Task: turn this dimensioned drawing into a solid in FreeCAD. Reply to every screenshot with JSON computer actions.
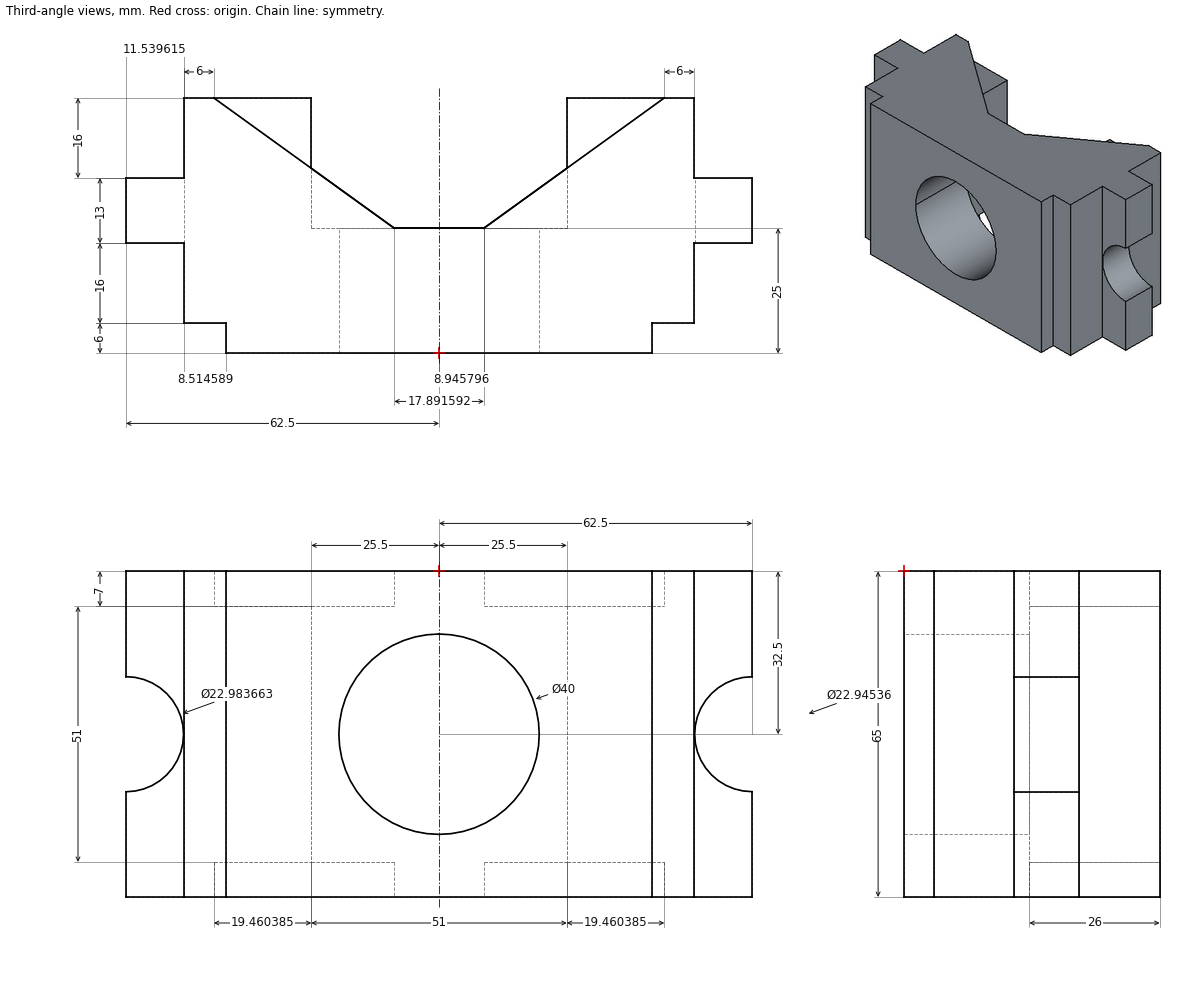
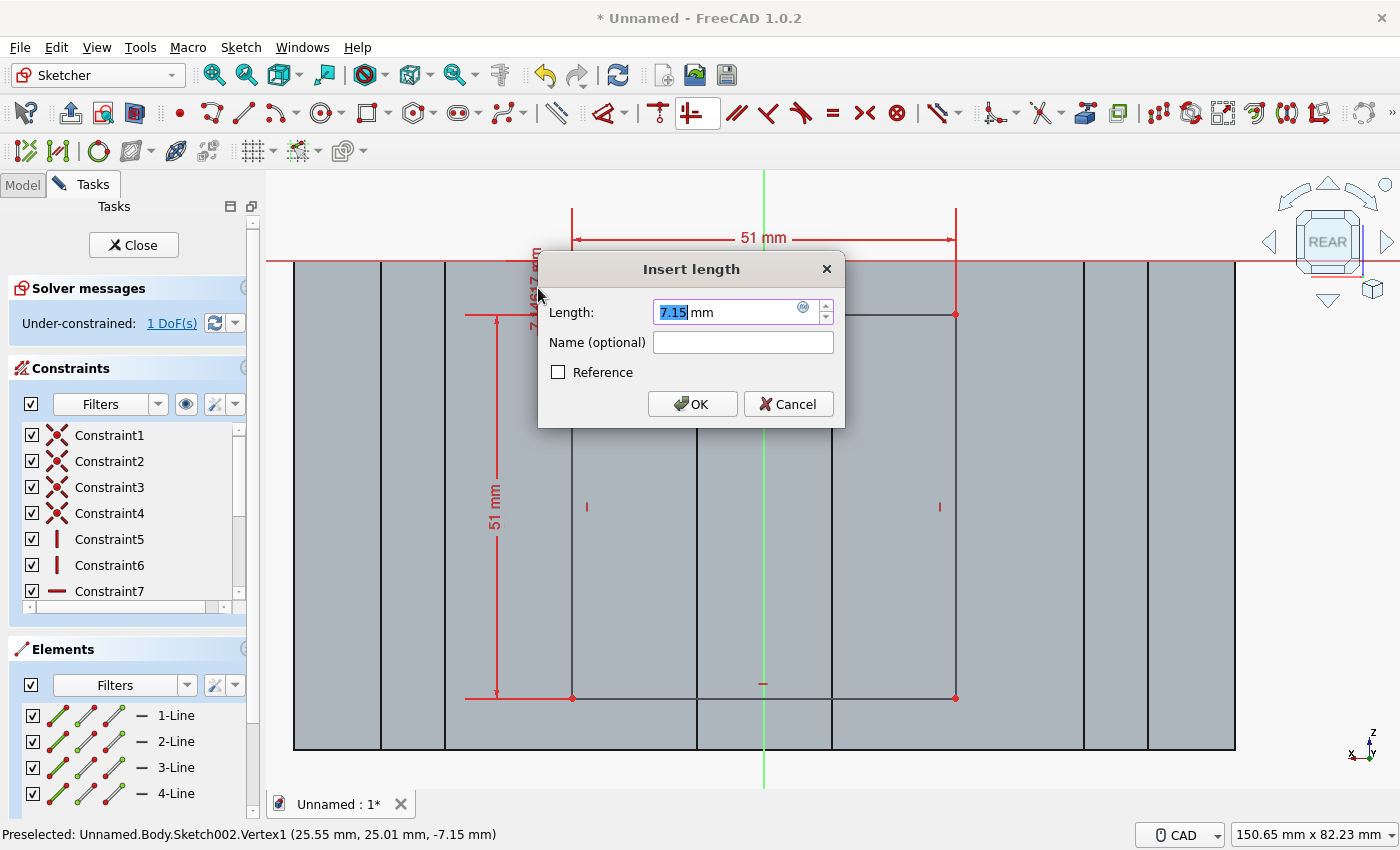
{"action": "type", "text": "7"}
{"action": "key", "text": "Return"}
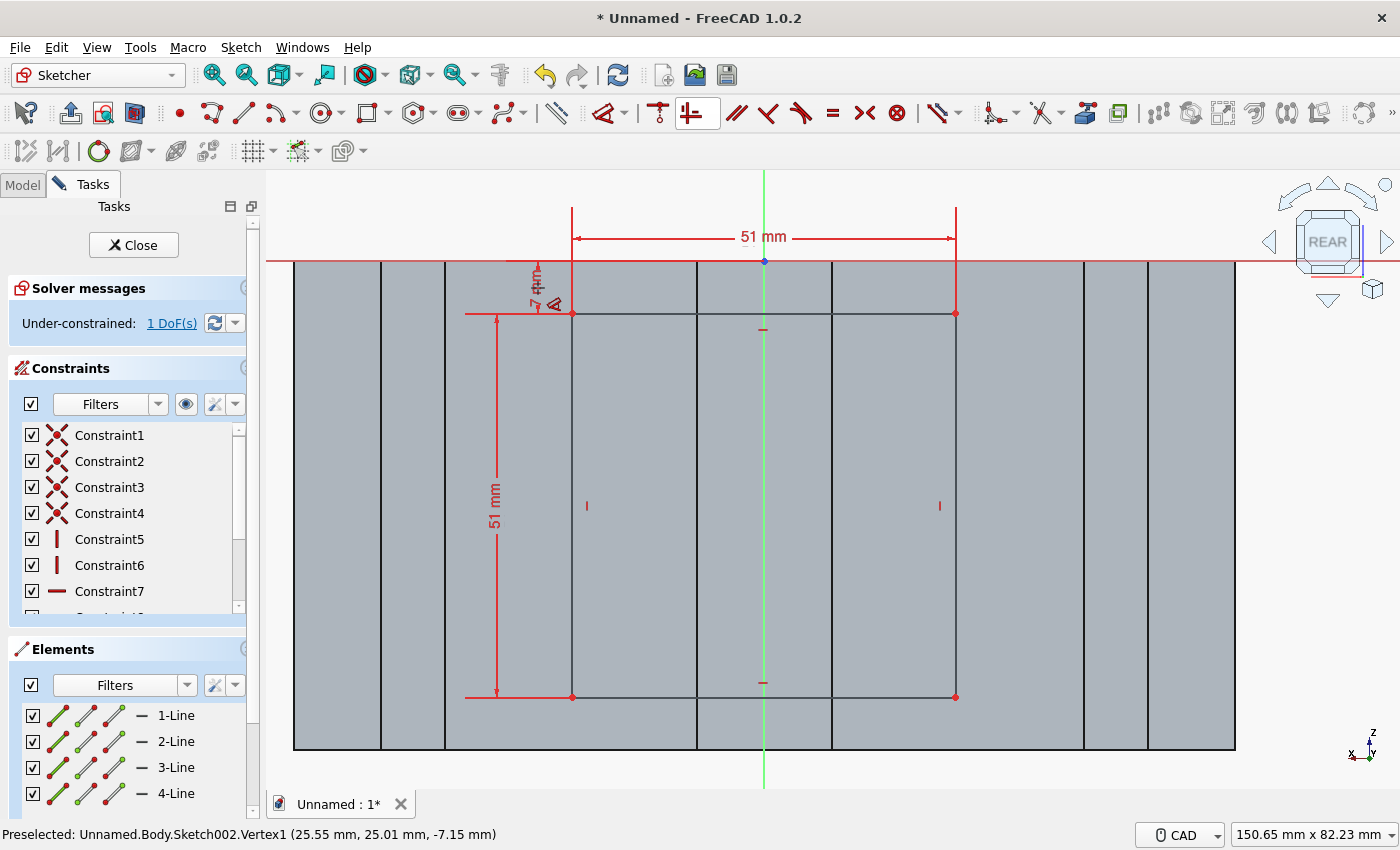
{"action": "left_click", "coordinate": [572, 314]}
{"action": "left_click", "coordinate": [668, 227]}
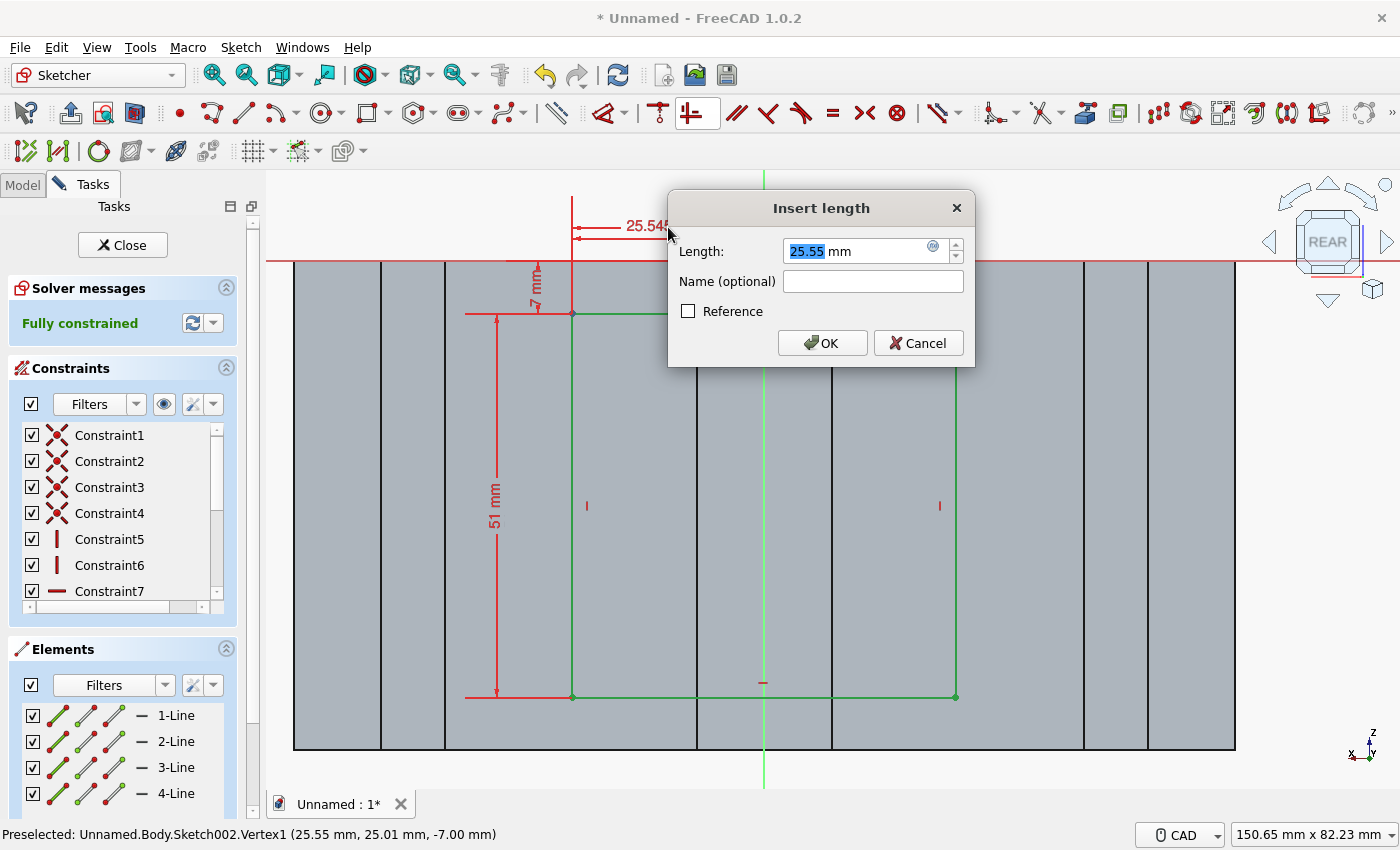
{"action": "type", "text": "25.5"}
{"action": "key", "text": "Return"}
{"action": "key", "text": "Escape"}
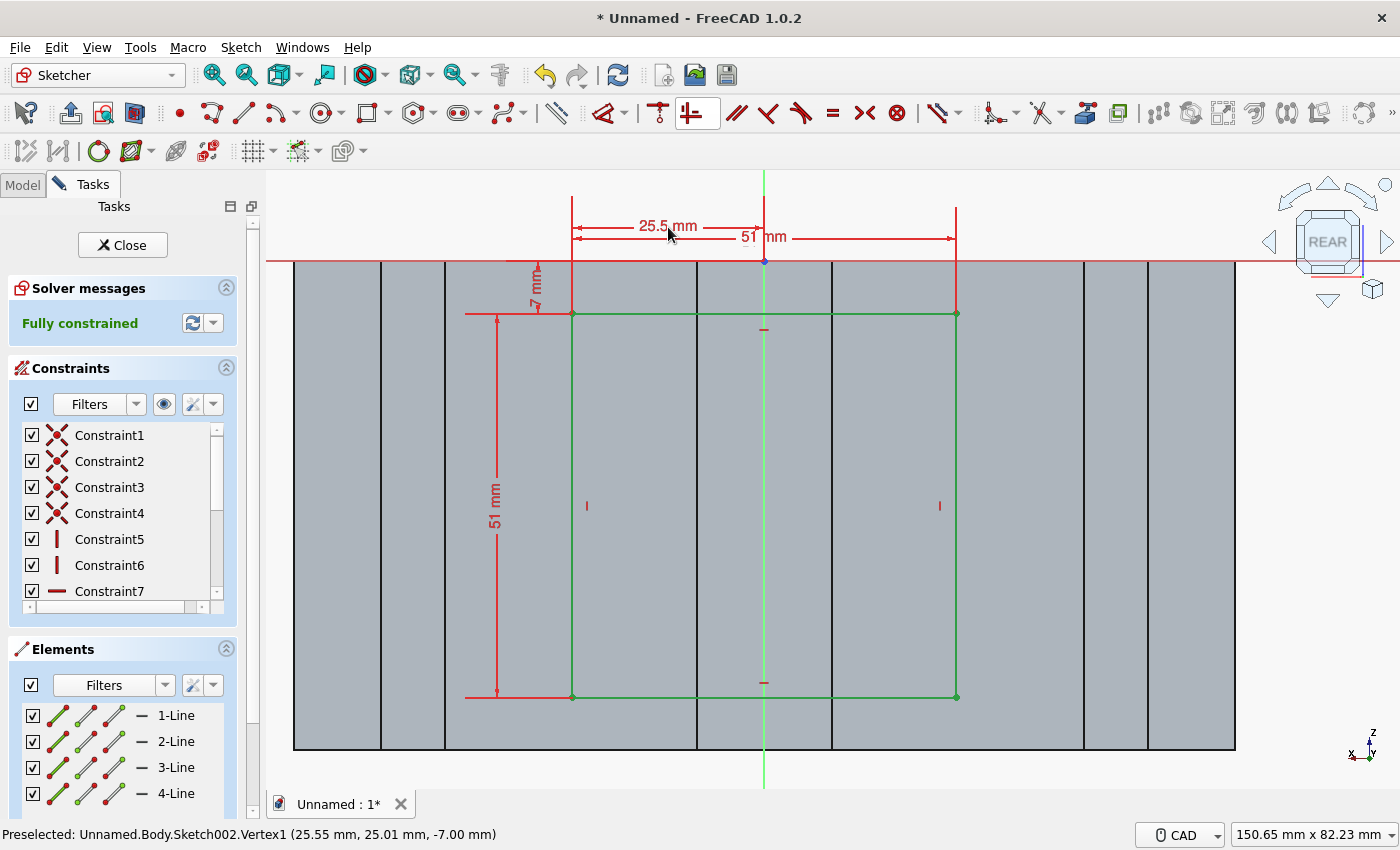
{"action": "left_click", "coordinate": [123, 245]}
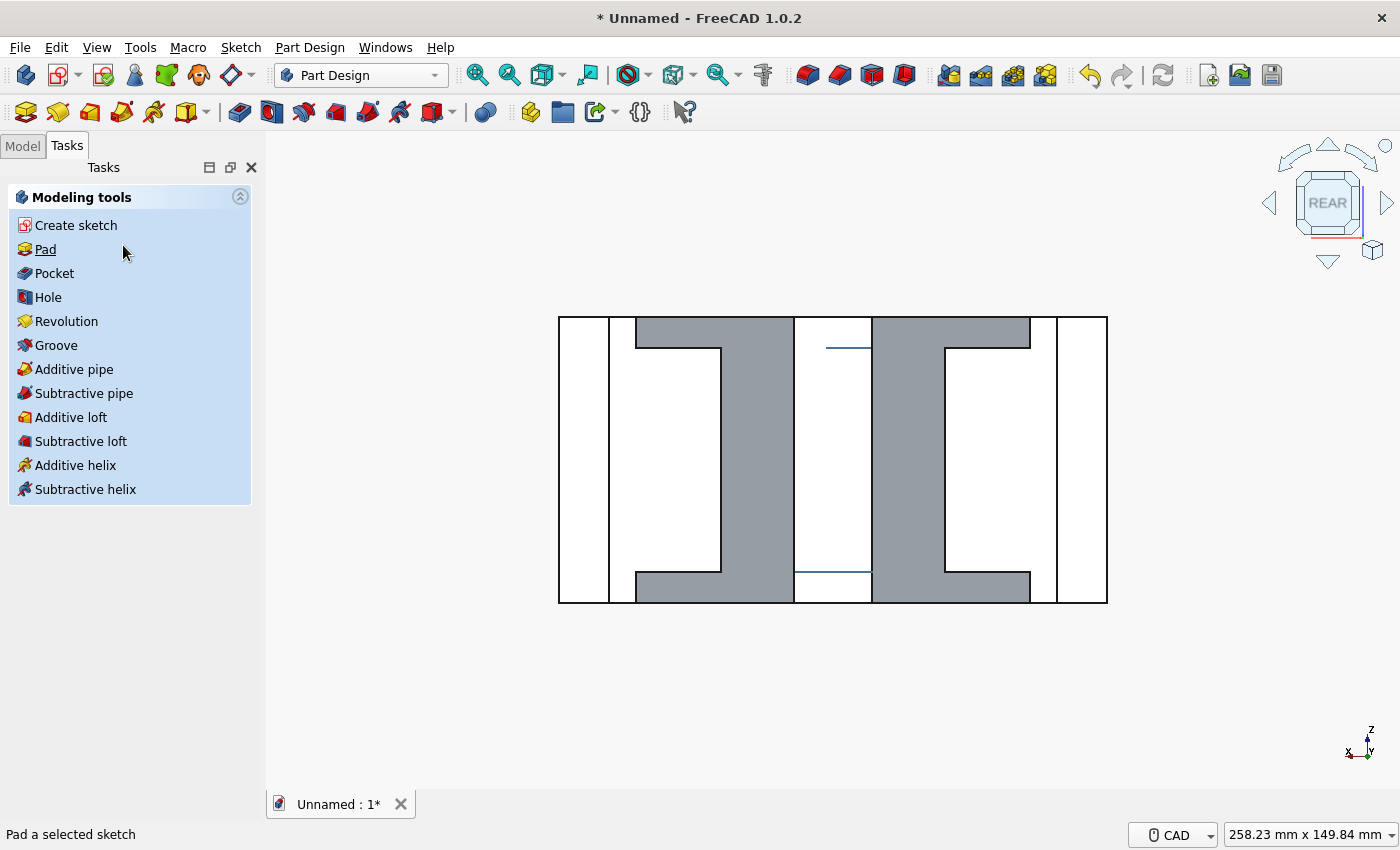
{"action": "left_click", "coordinate": [240, 112]}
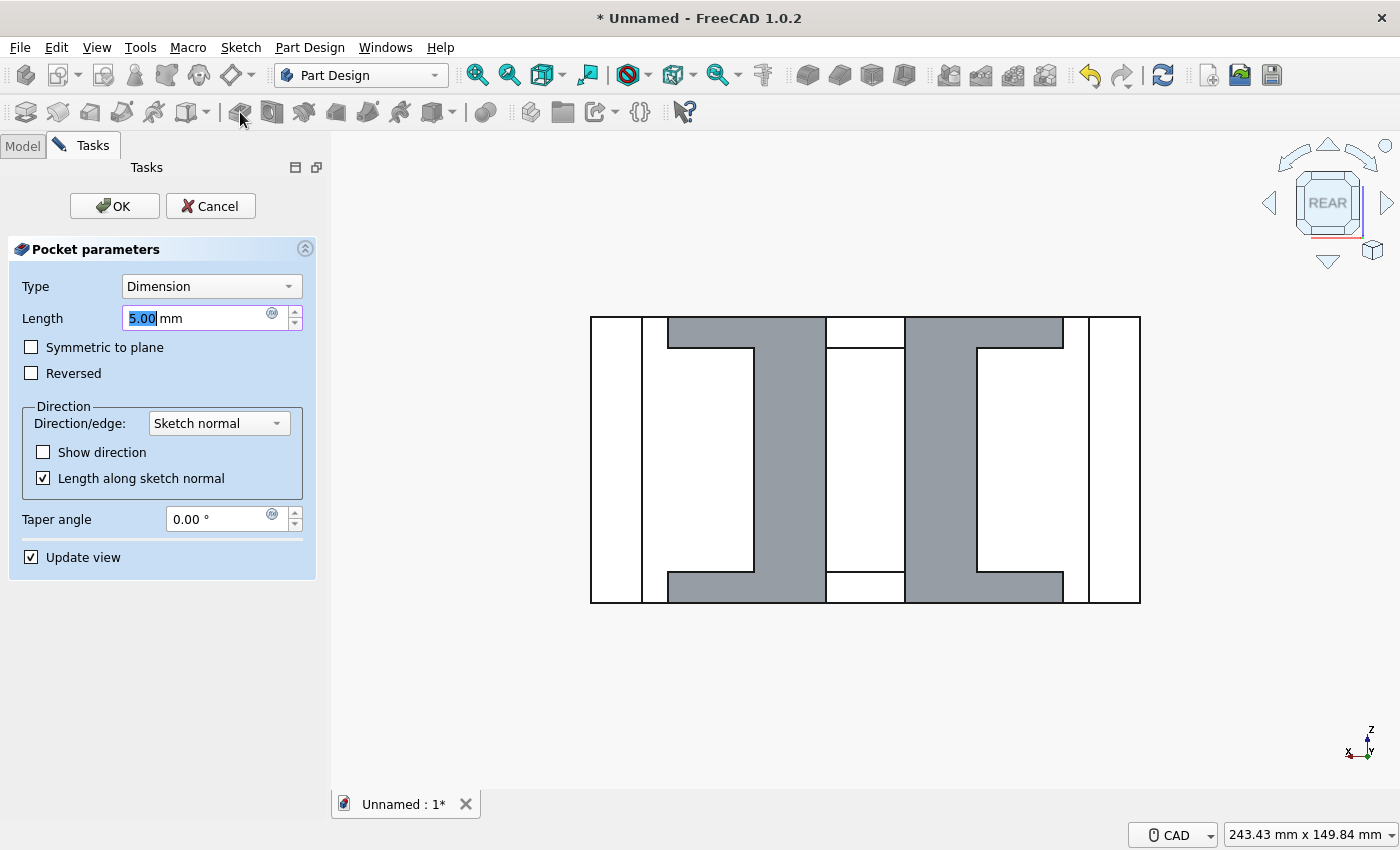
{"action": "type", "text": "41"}
{"action": "key", "text": "Tab"}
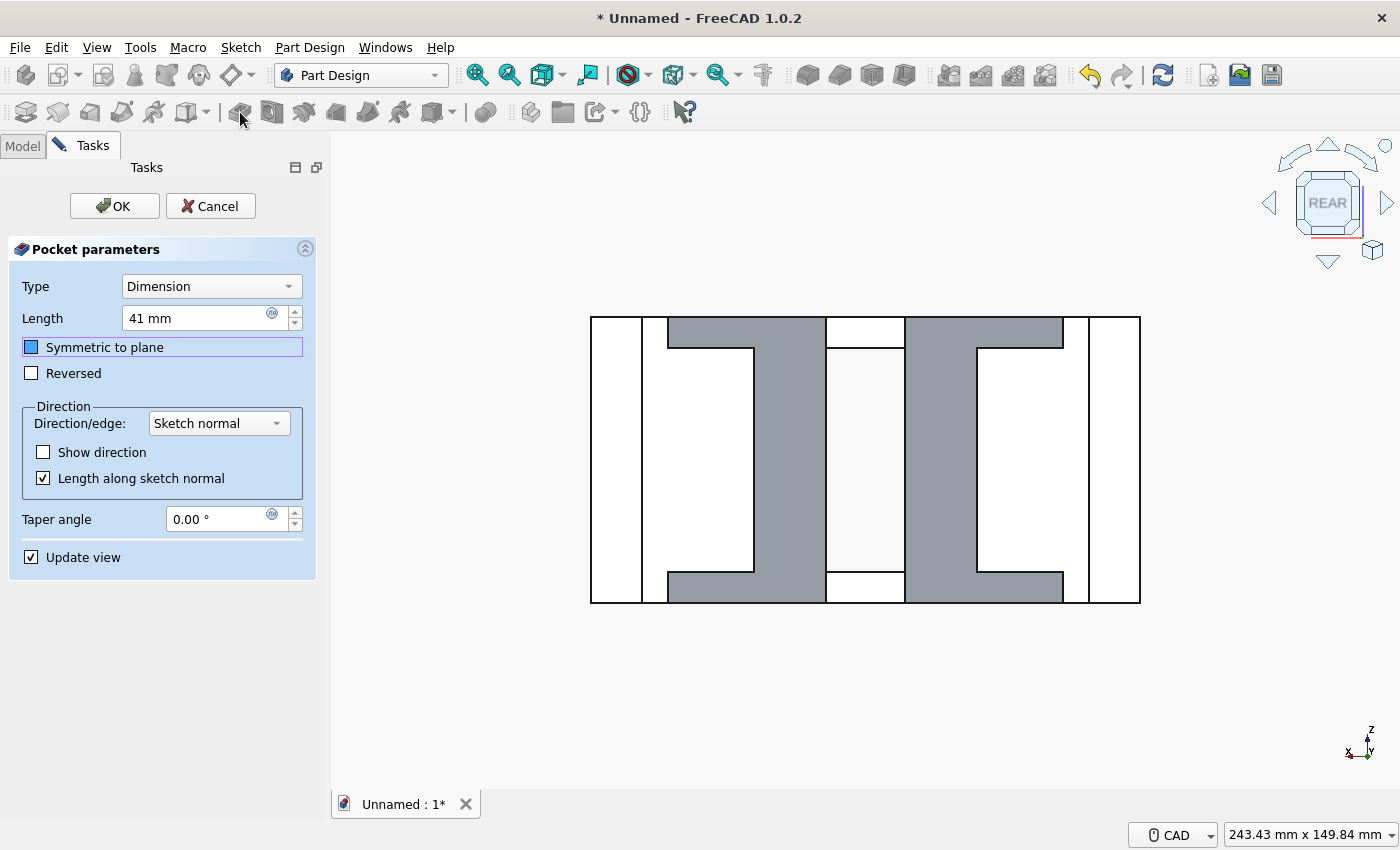
{"action": "left_click", "coordinate": [30, 373]}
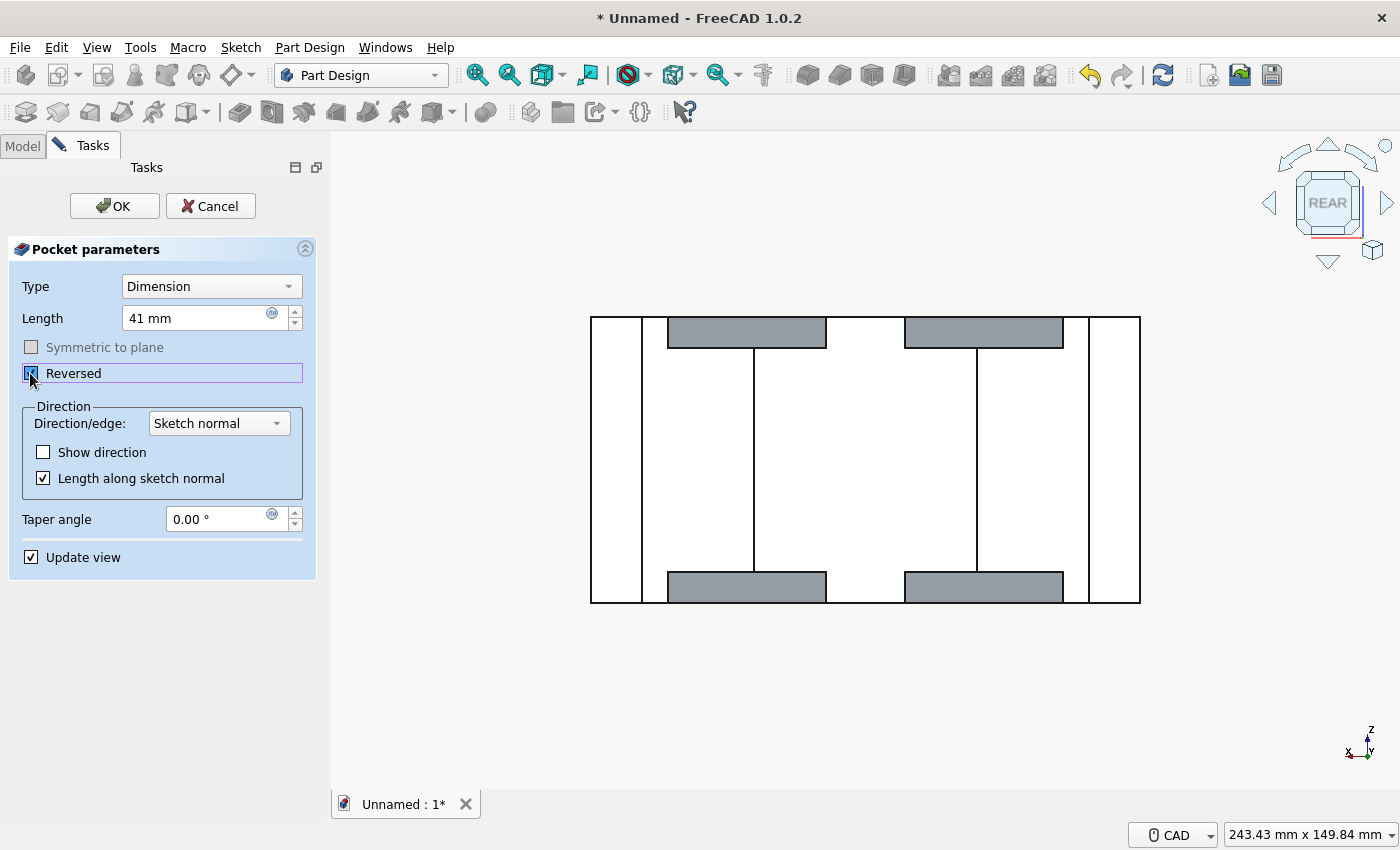
{"action": "left_click", "coordinate": [115, 206]}